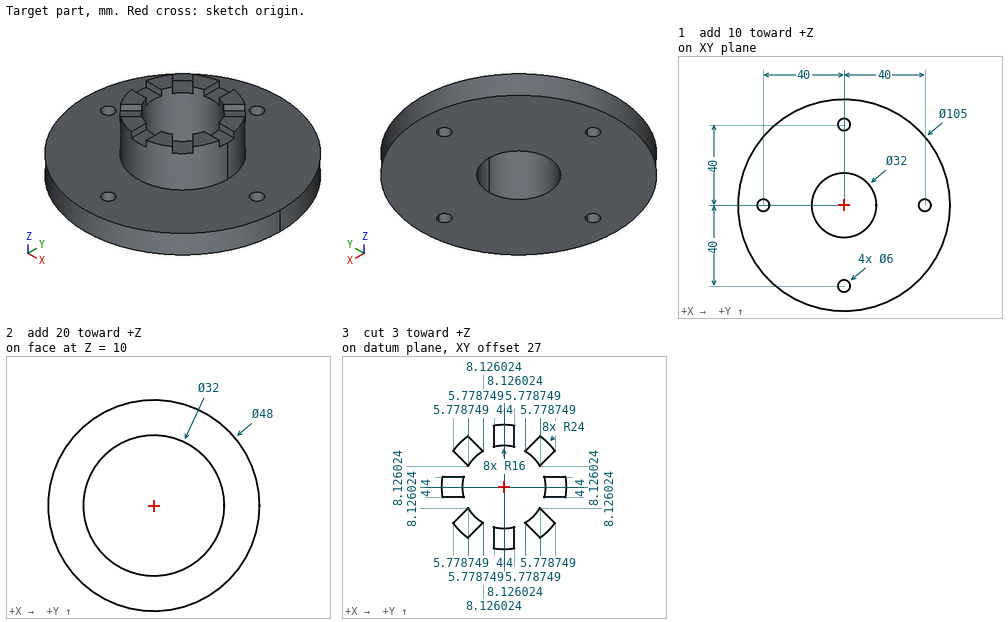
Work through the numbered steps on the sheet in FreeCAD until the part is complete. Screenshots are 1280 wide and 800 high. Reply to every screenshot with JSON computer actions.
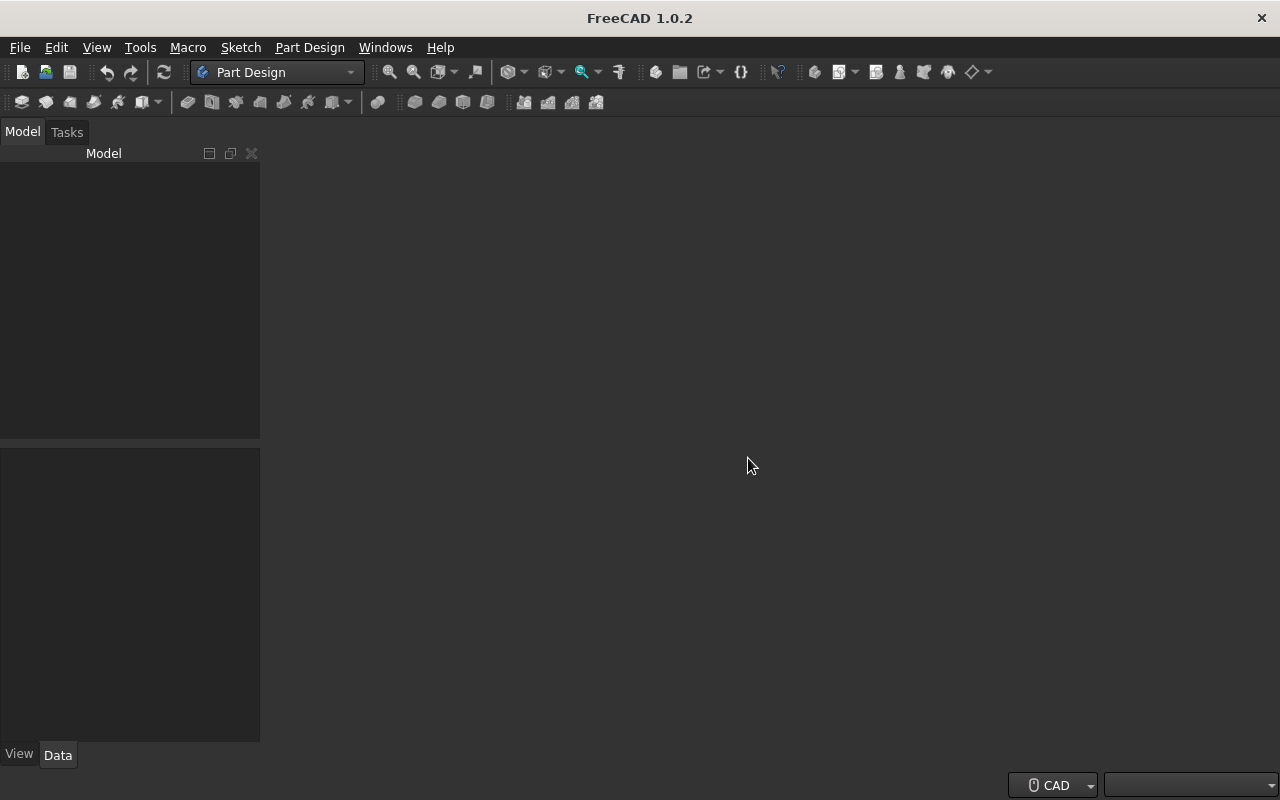
{"action": "left_click", "coordinate": [22, 72]}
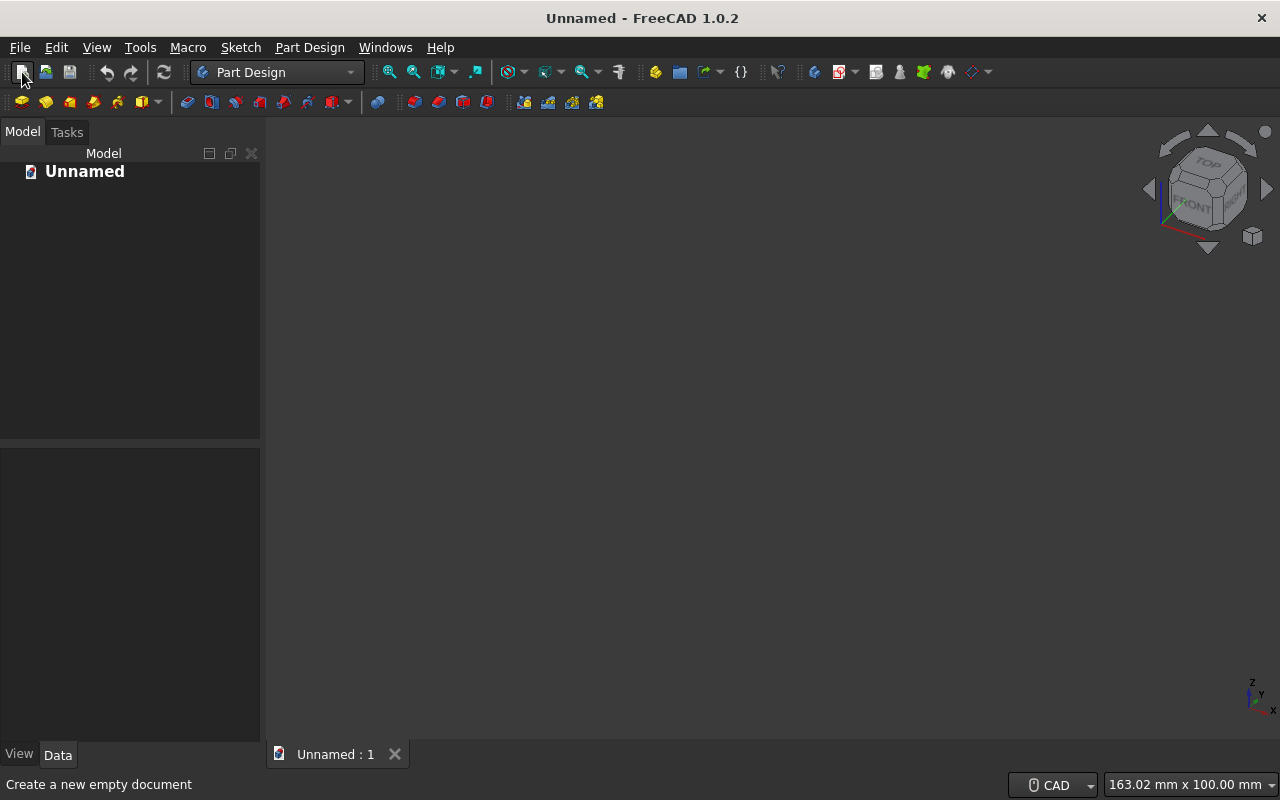
{"action": "left_click", "coordinate": [840, 72]}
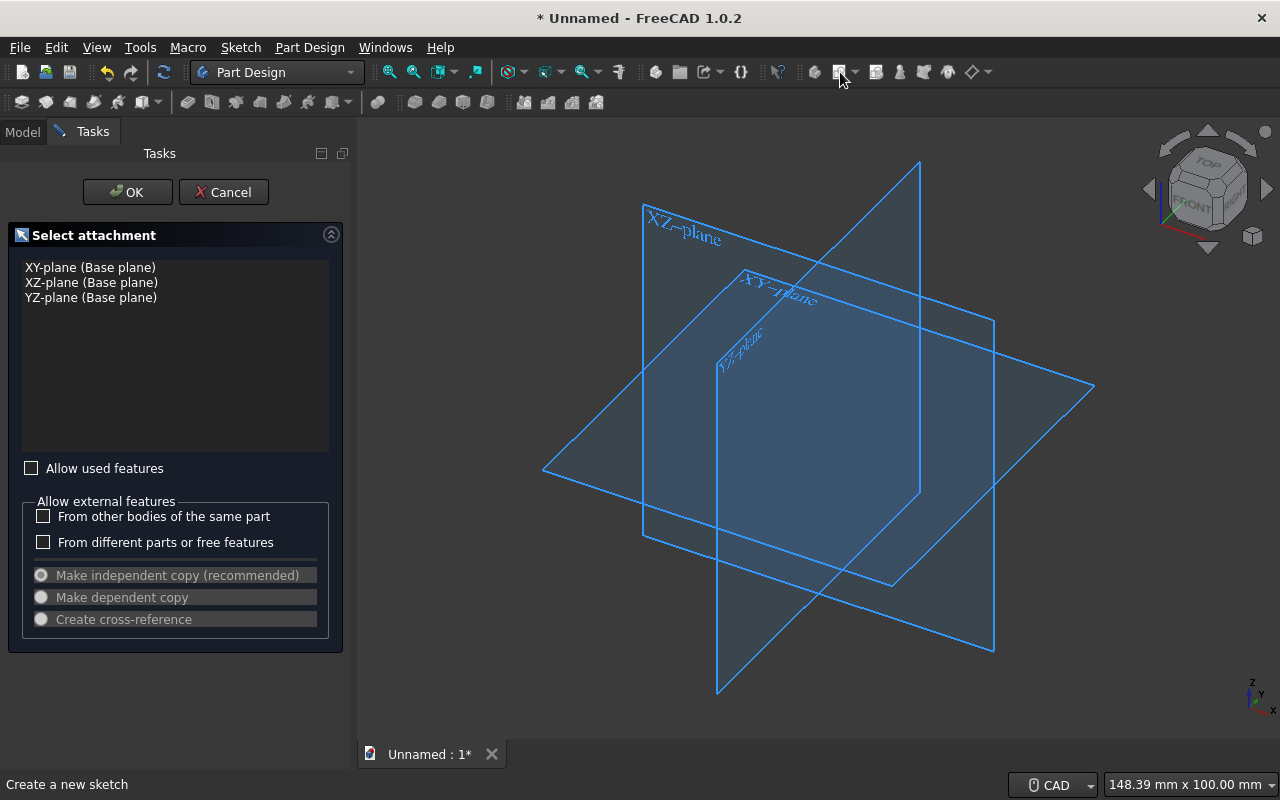
{"action": "left_click", "coordinate": [82, 268]}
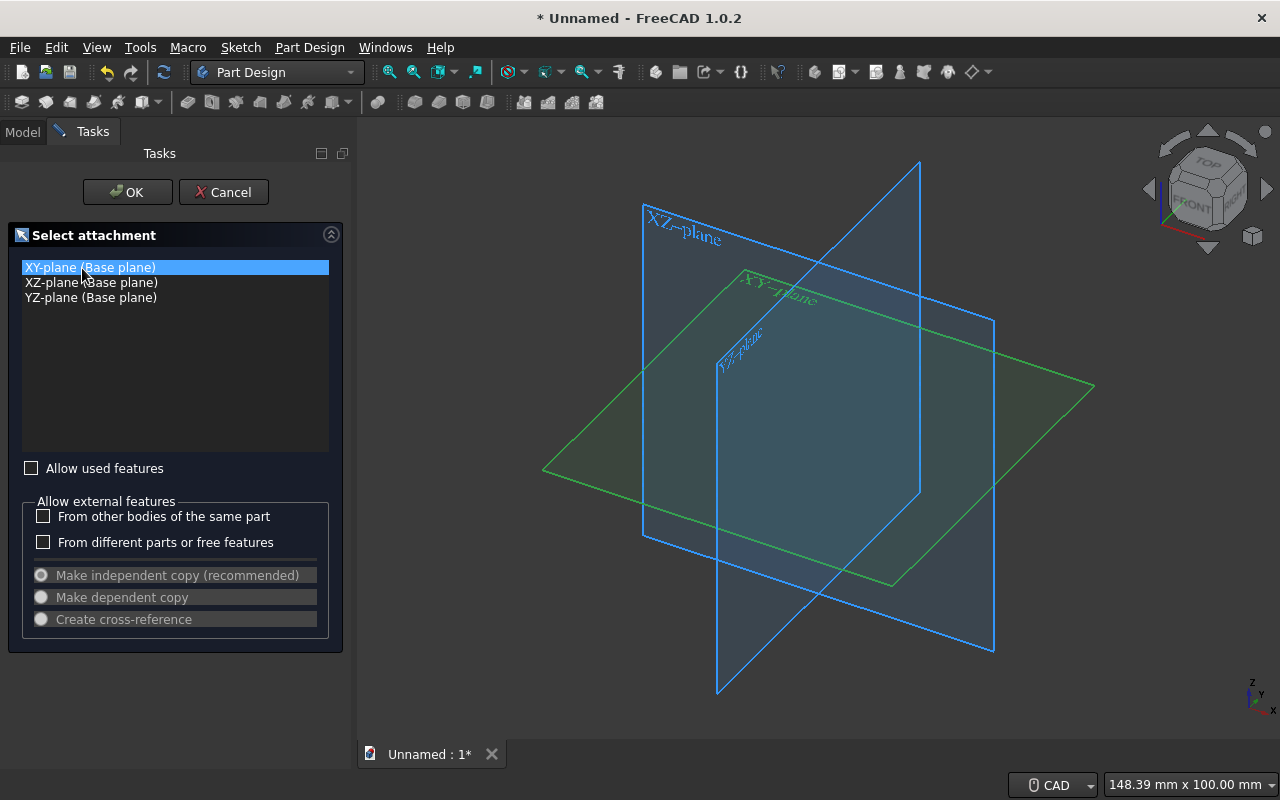
{"action": "left_click", "coordinate": [128, 192]}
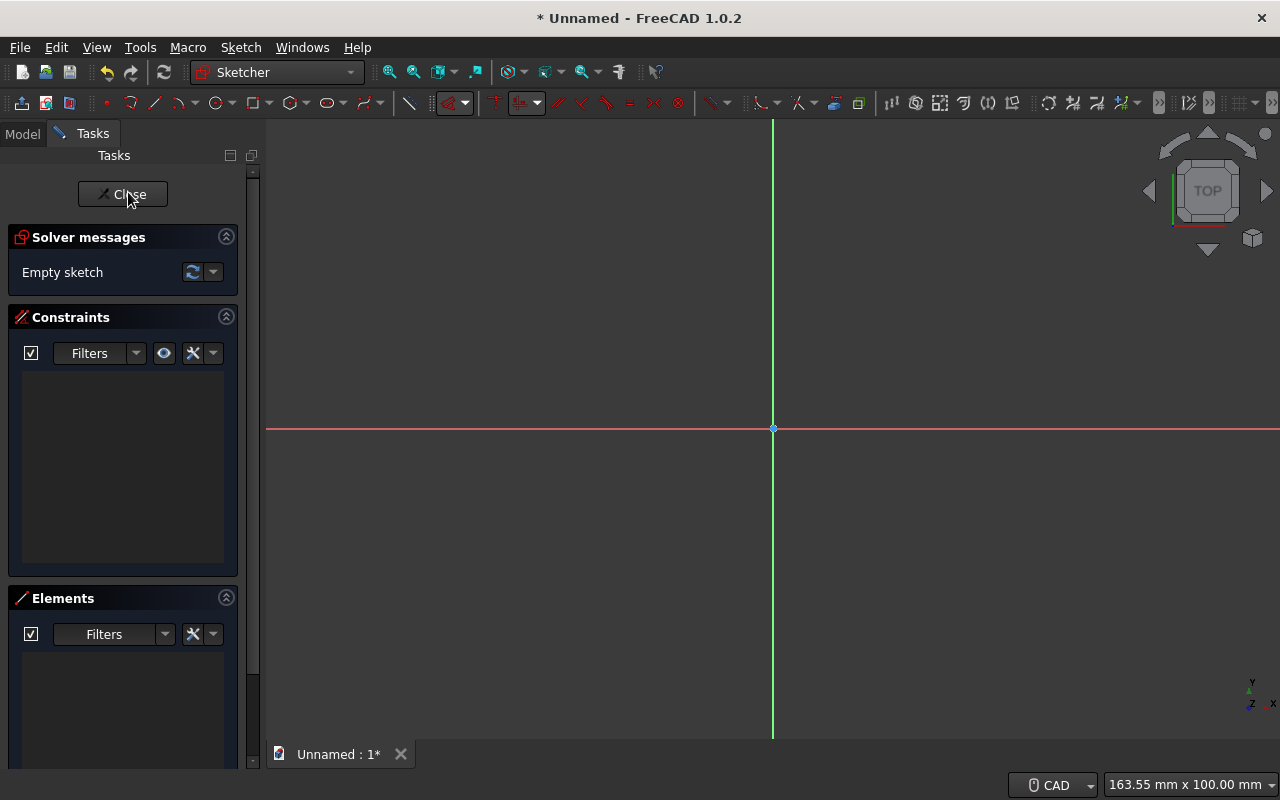
{"action": "scroll", "coordinate": [565, 429], "scroll_direction": "down", "scroll_amount": 2}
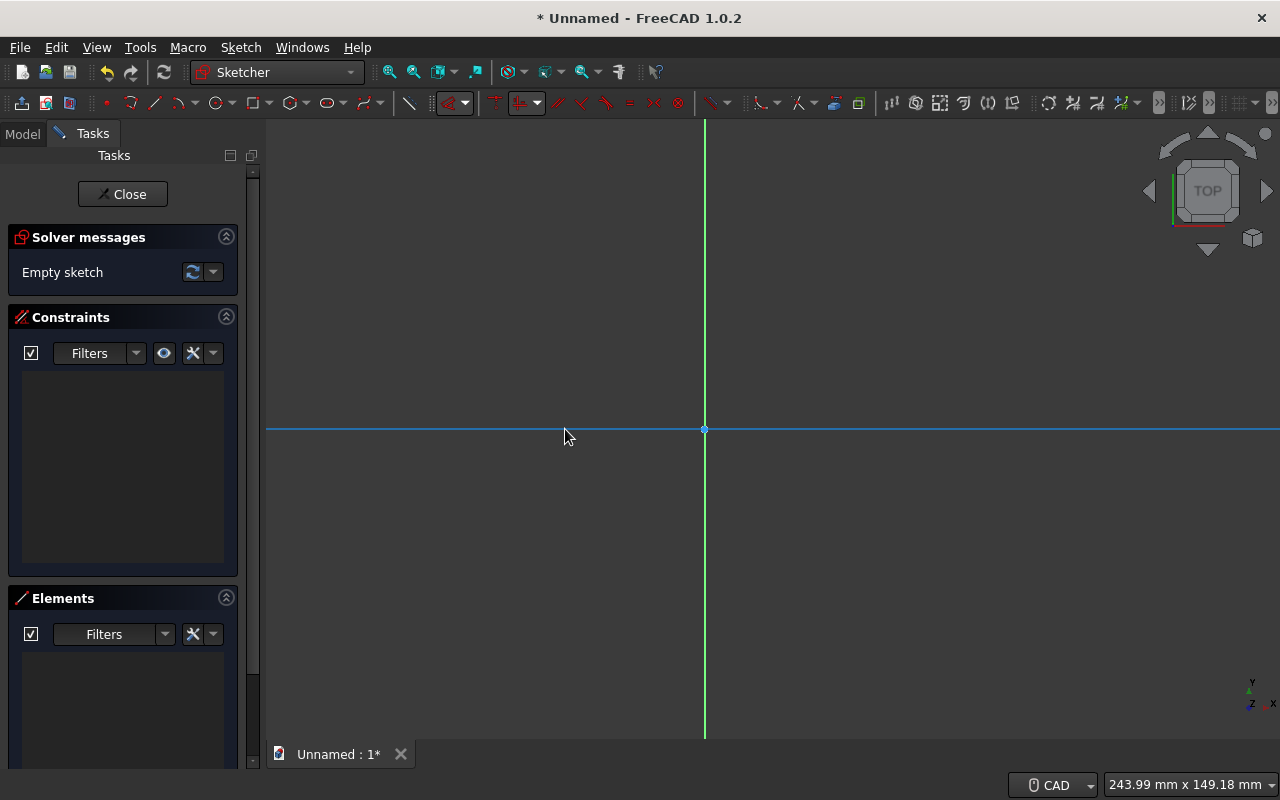
{"action": "left_click", "coordinate": [216, 104]}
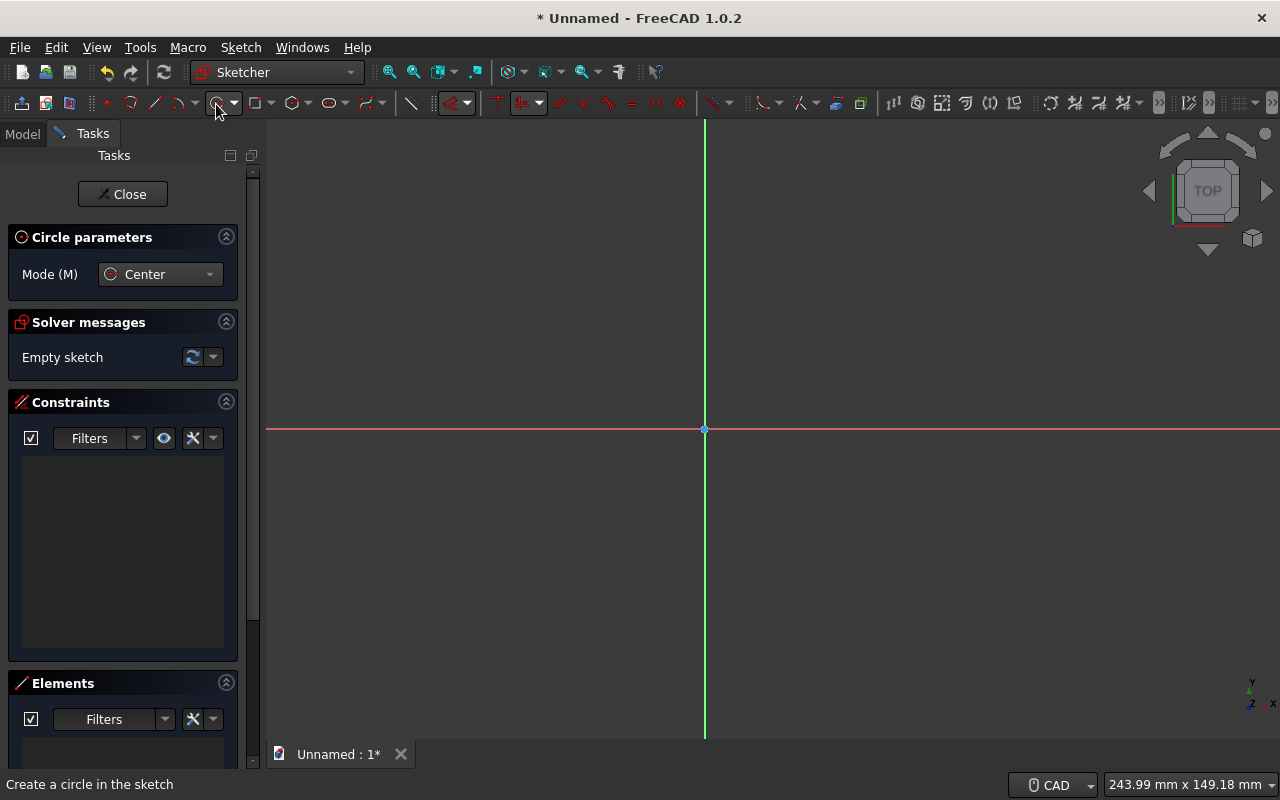
{"action": "left_click", "coordinate": [705, 429]}
{"action": "left_click", "coordinate": [859, 275]}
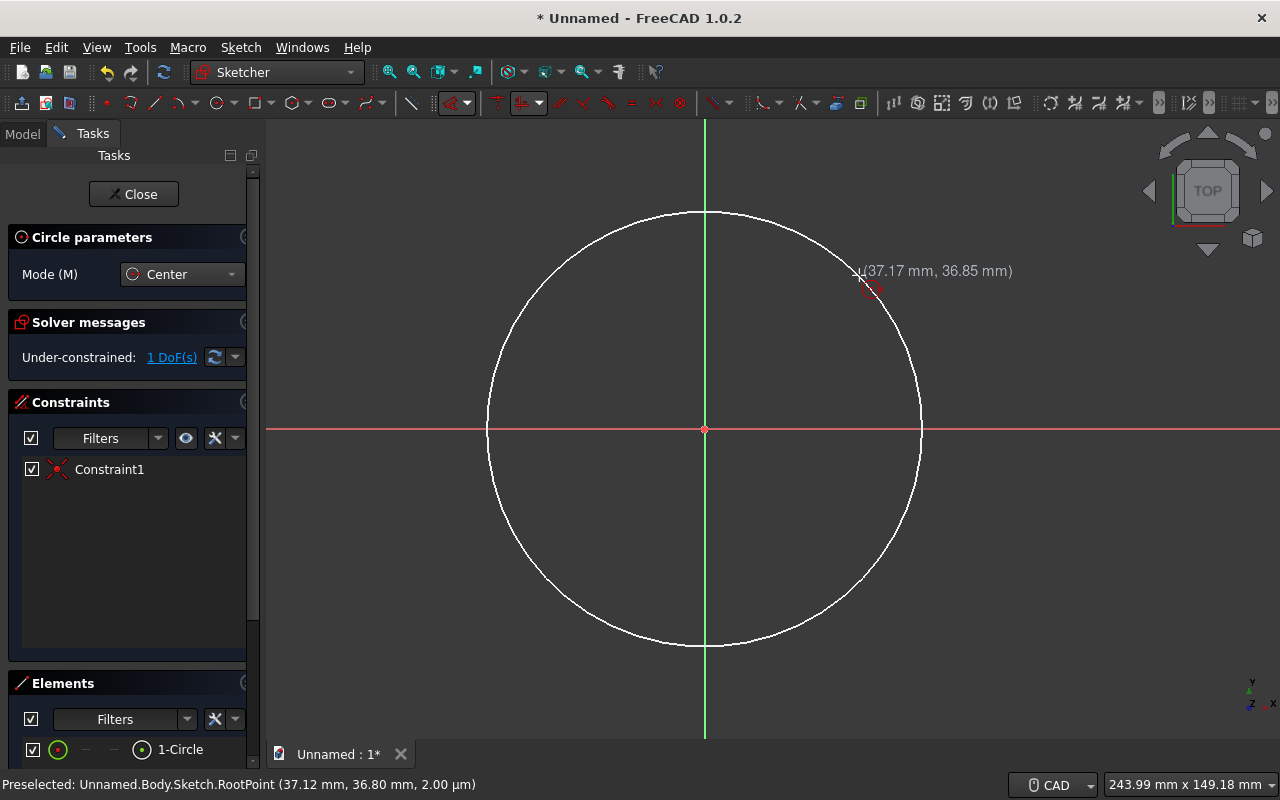
{"action": "scroll", "coordinate": [705, 595], "scroll_direction": "up", "scroll_amount": 3}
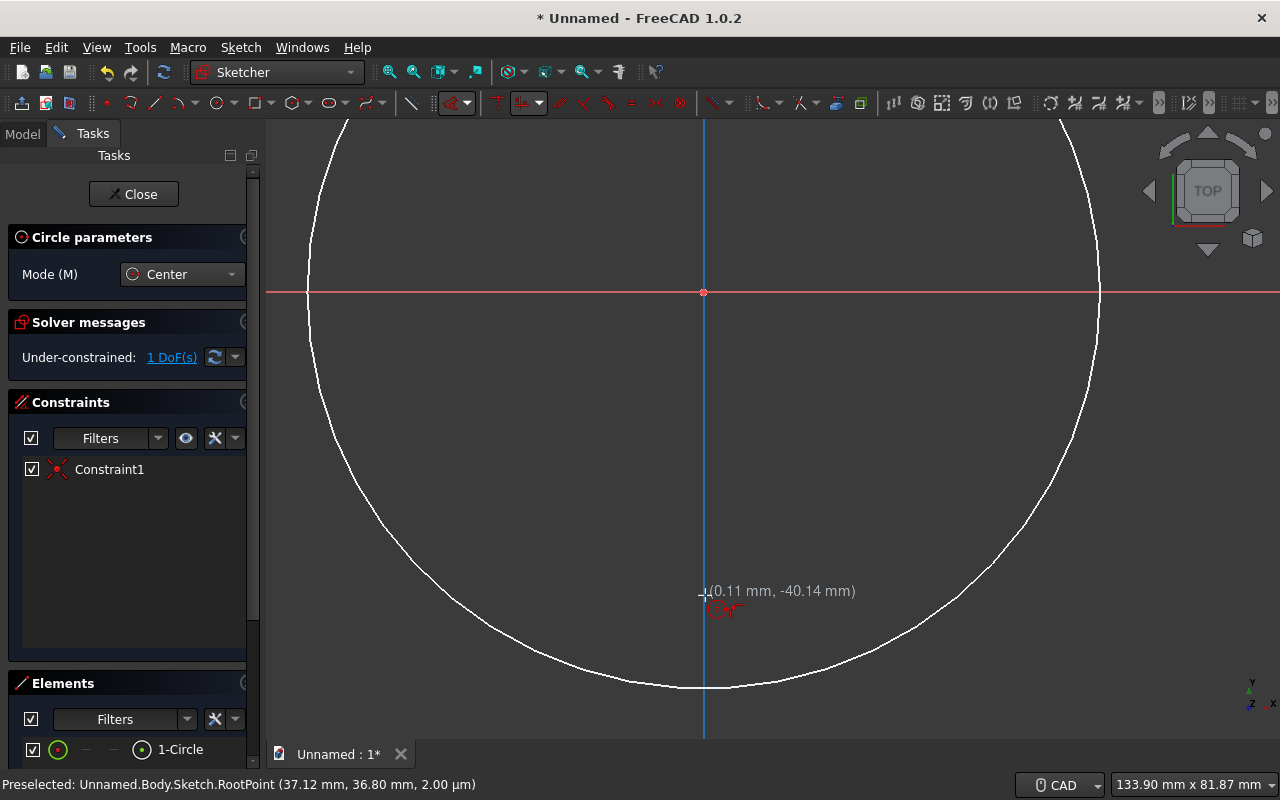
{"action": "left_click", "coordinate": [704, 595]}
{"action": "left_click", "coordinate": [720, 579]}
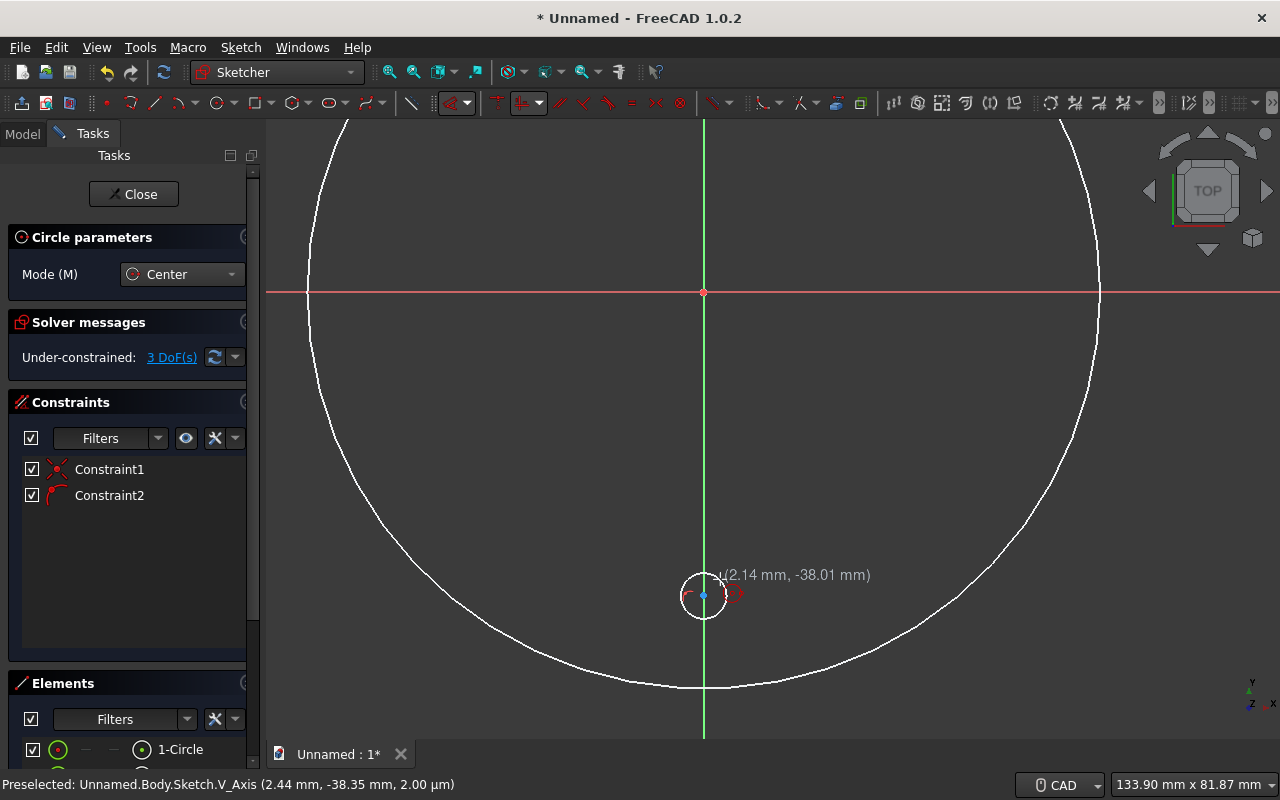
{"action": "left_click", "coordinate": [401, 292]}
{"action": "left_click", "coordinate": [417, 276]}